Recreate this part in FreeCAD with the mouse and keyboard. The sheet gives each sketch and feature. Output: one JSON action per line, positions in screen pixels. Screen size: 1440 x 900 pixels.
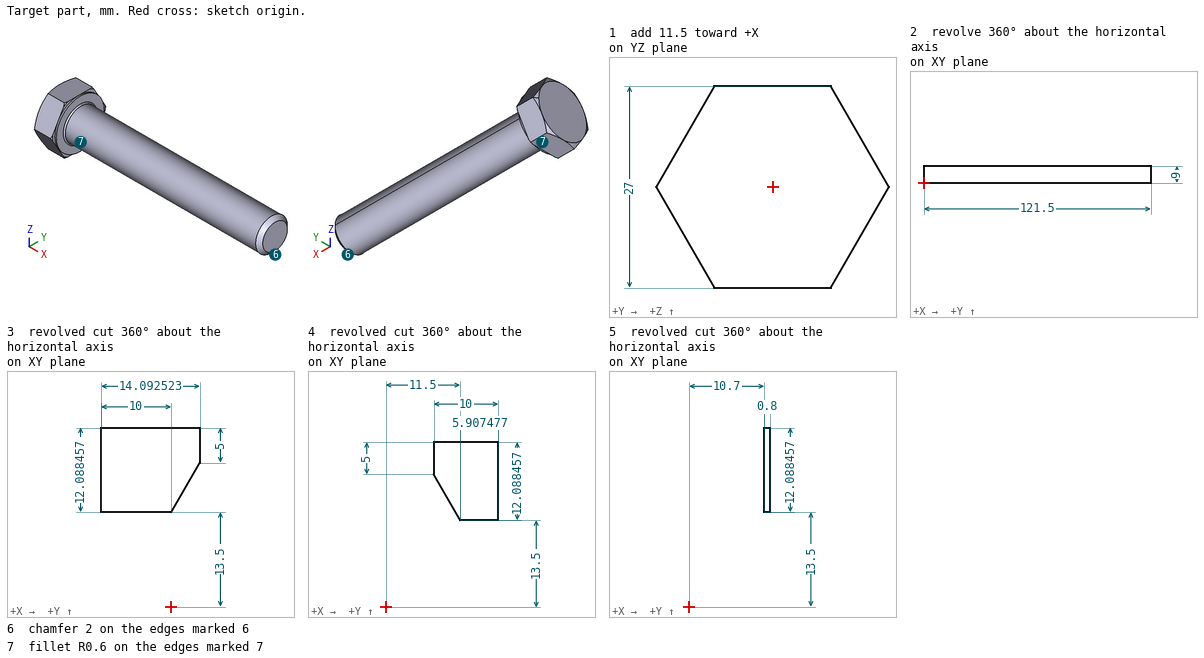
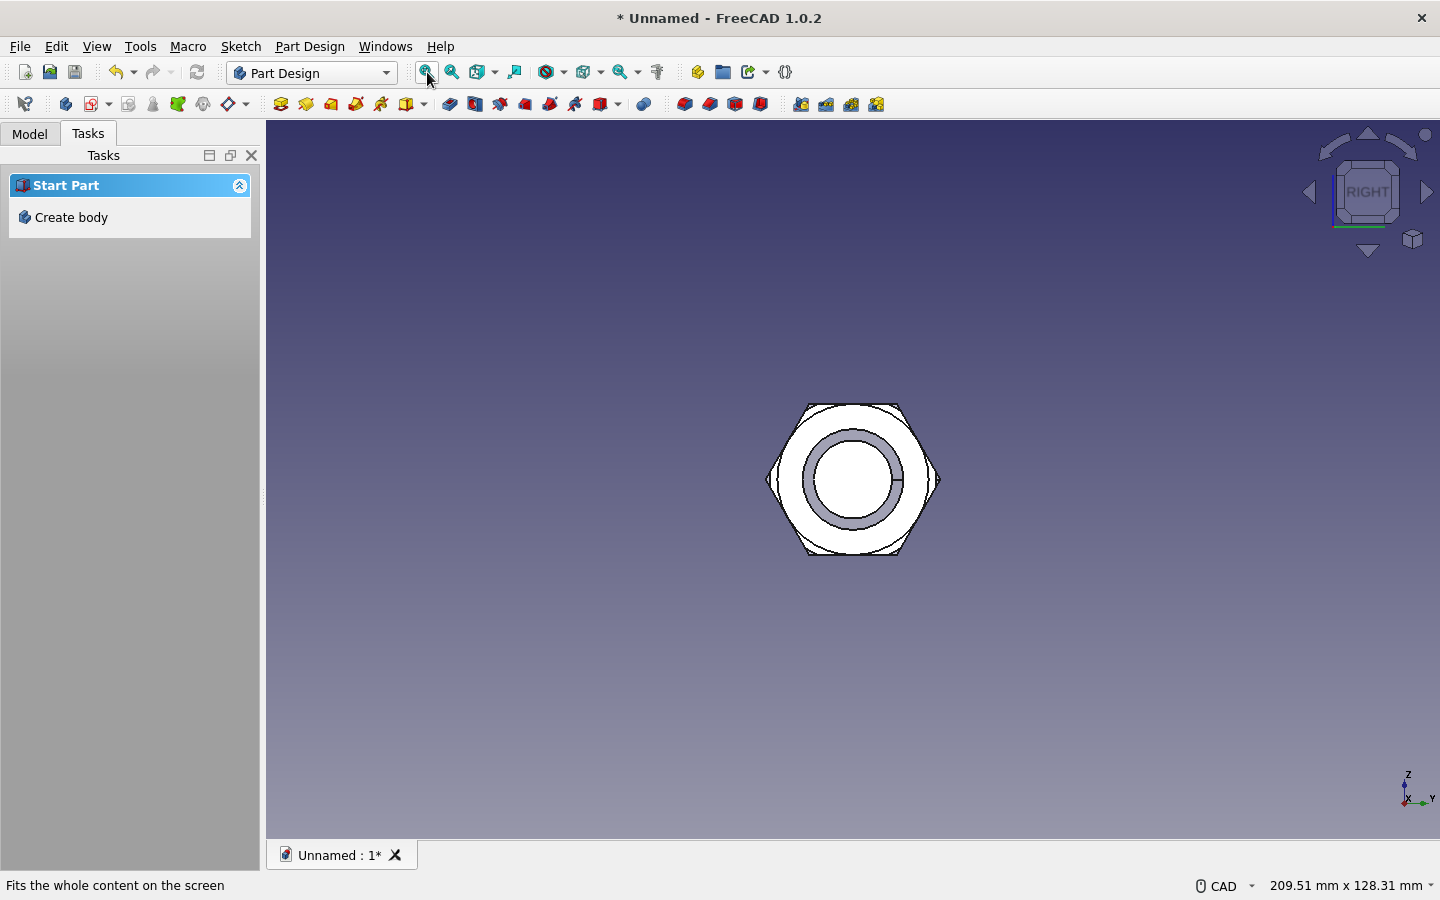
{"action": "key", "text": "5"}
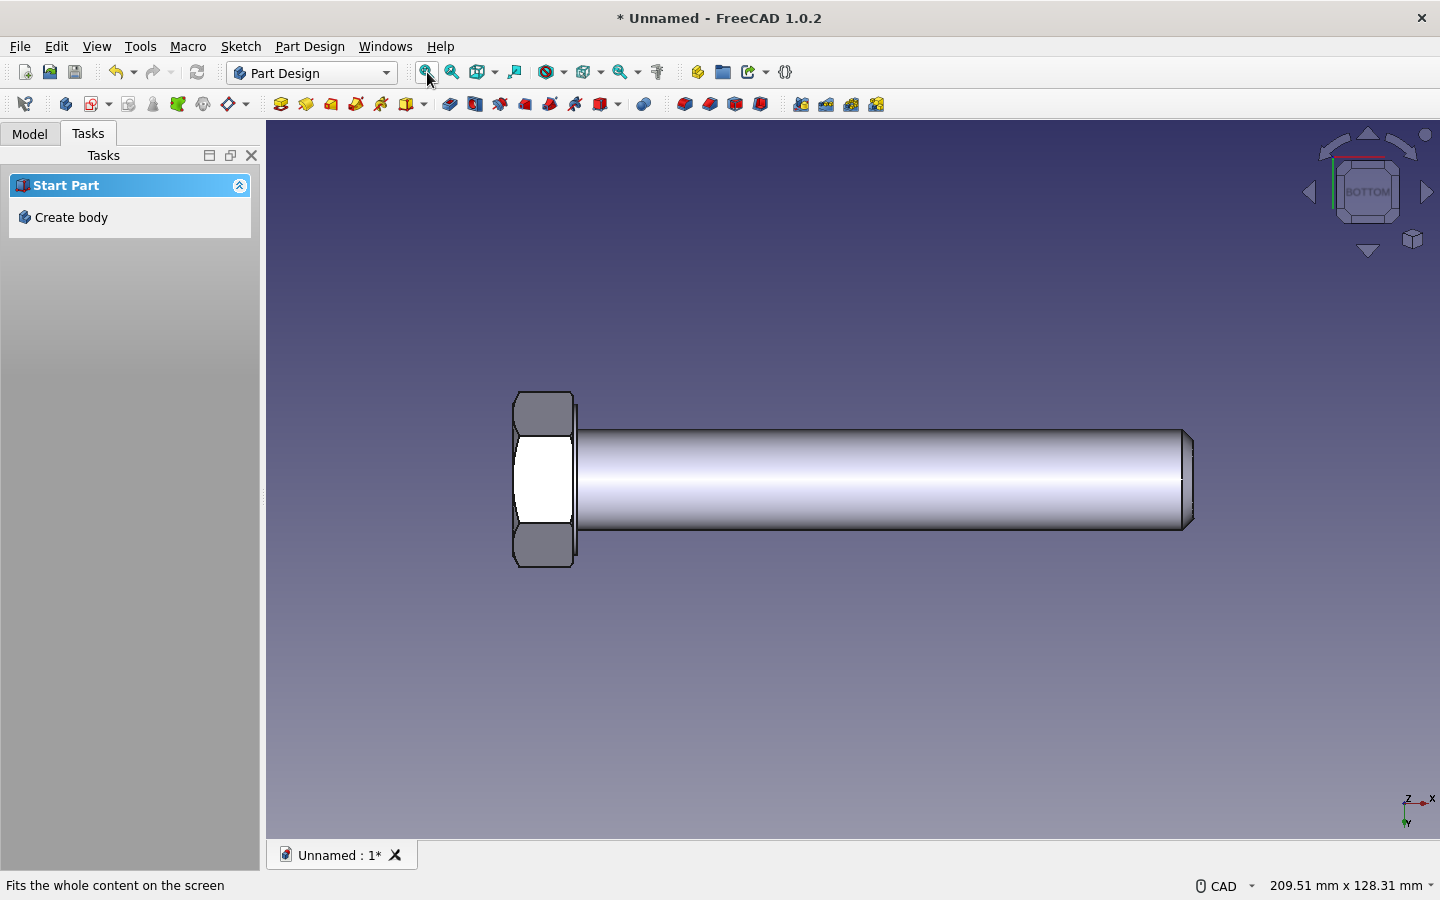
{"action": "key", "text": "4"}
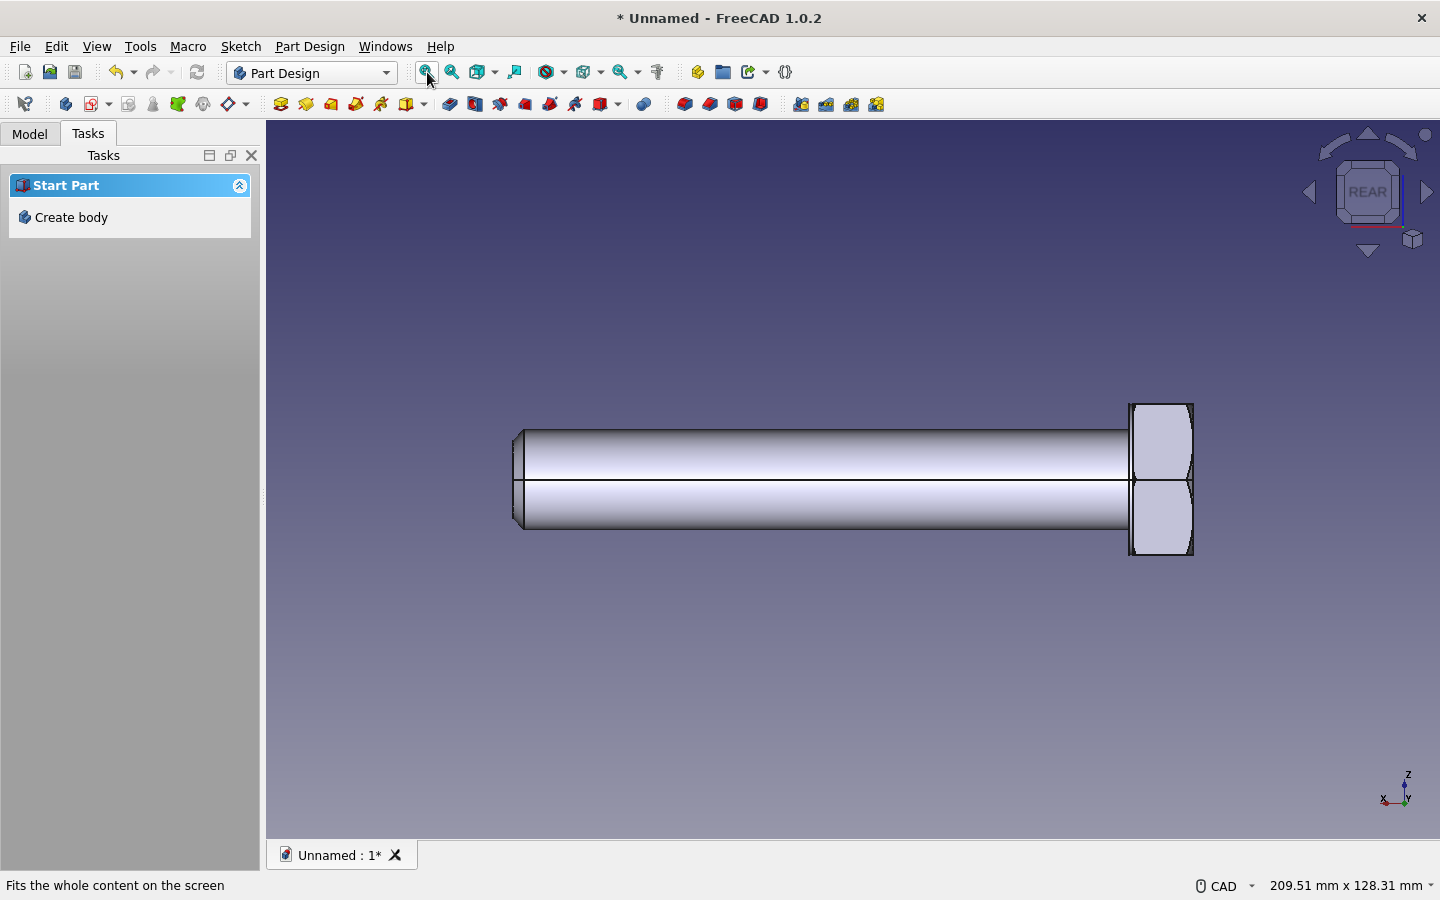
{"action": "key", "text": "6"}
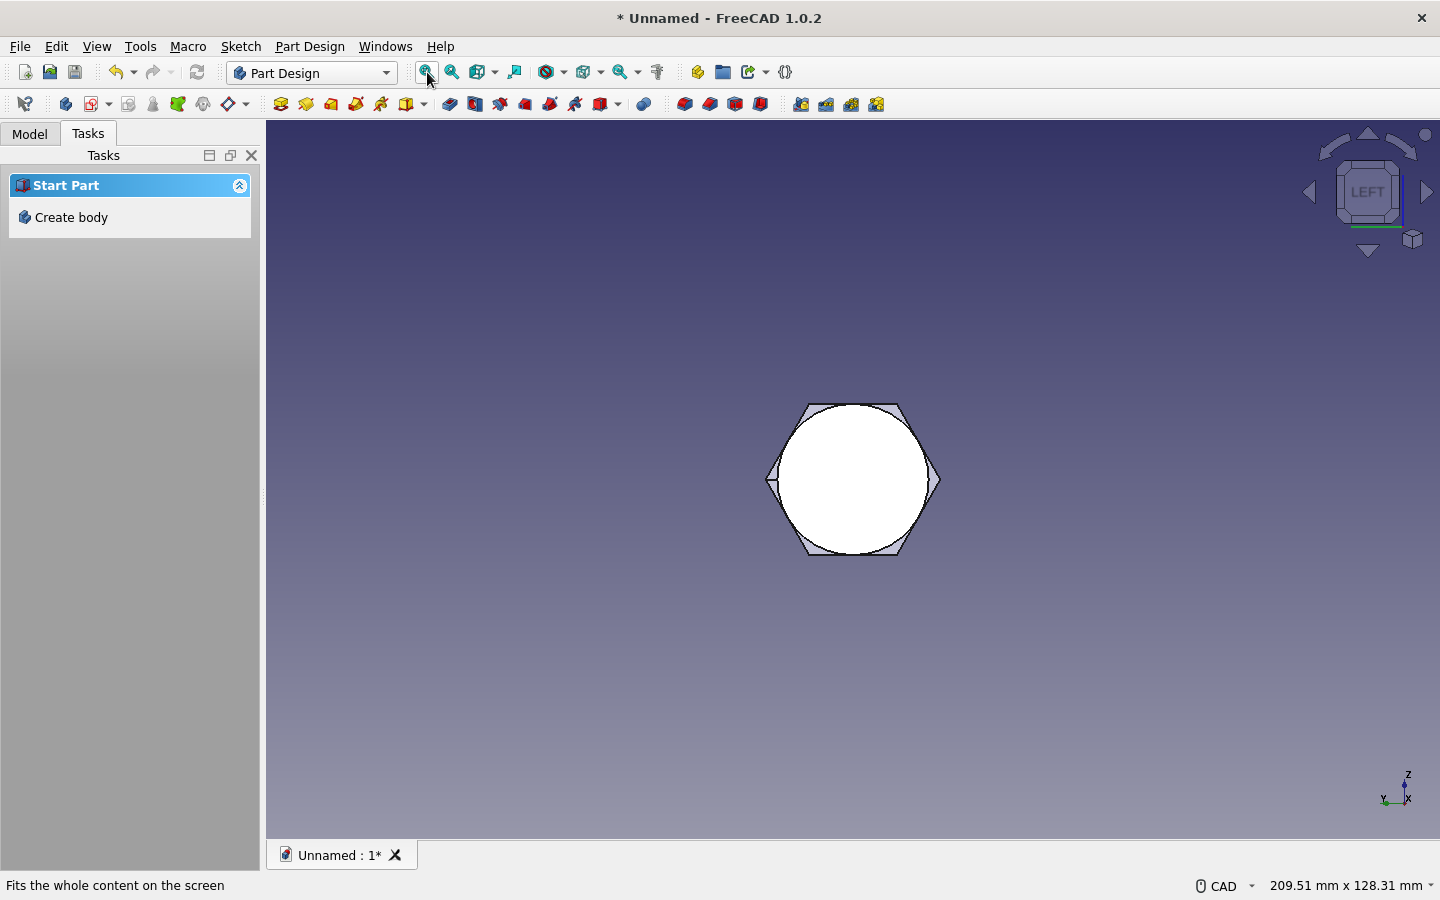
{"action": "left_click", "coordinate": [427, 72]}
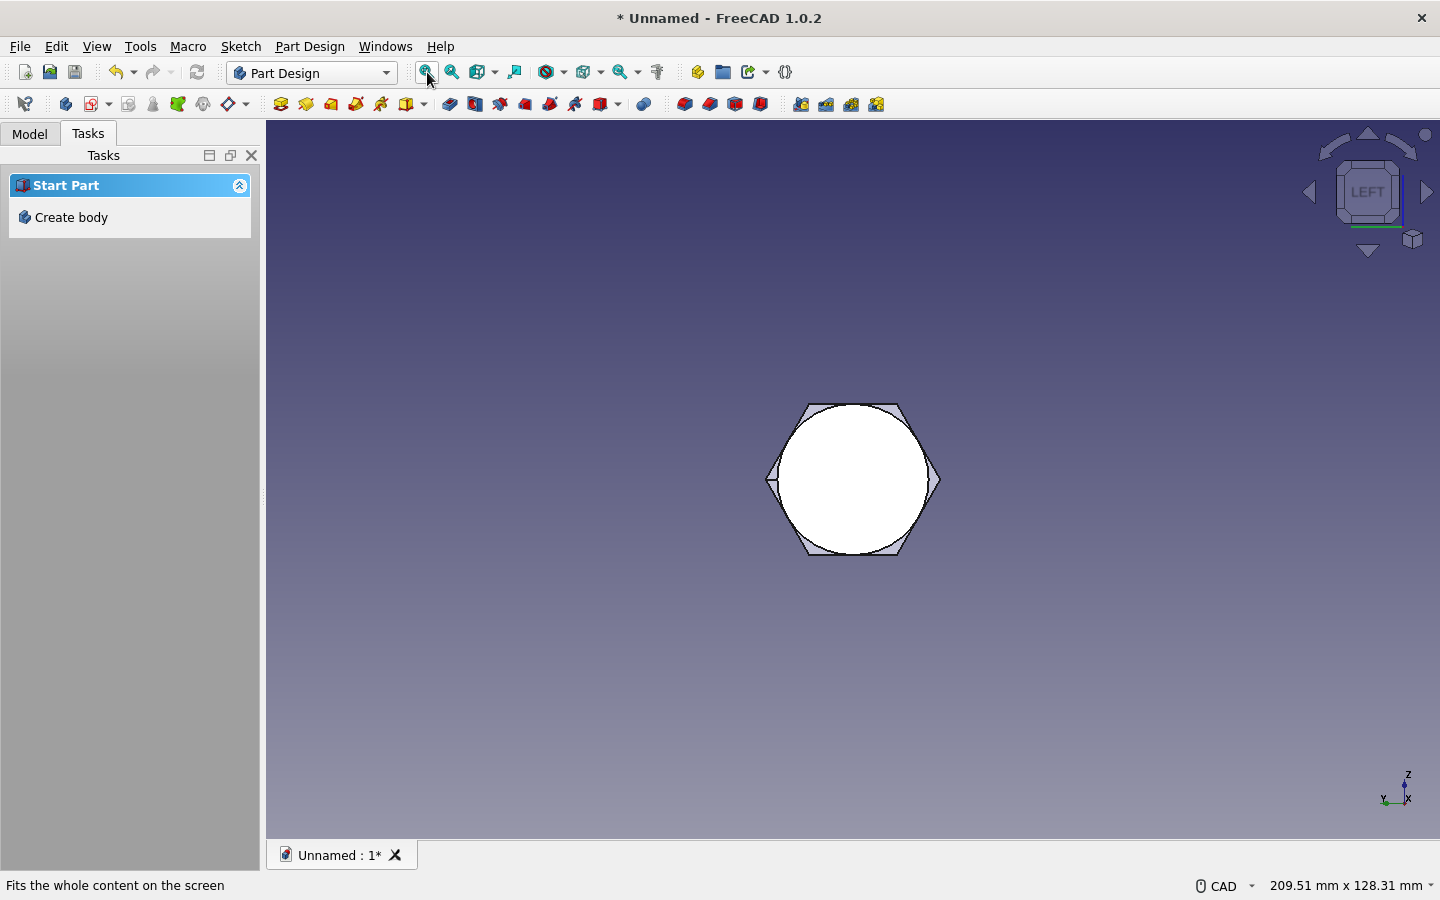
{"action": "key", "text": "v 3"}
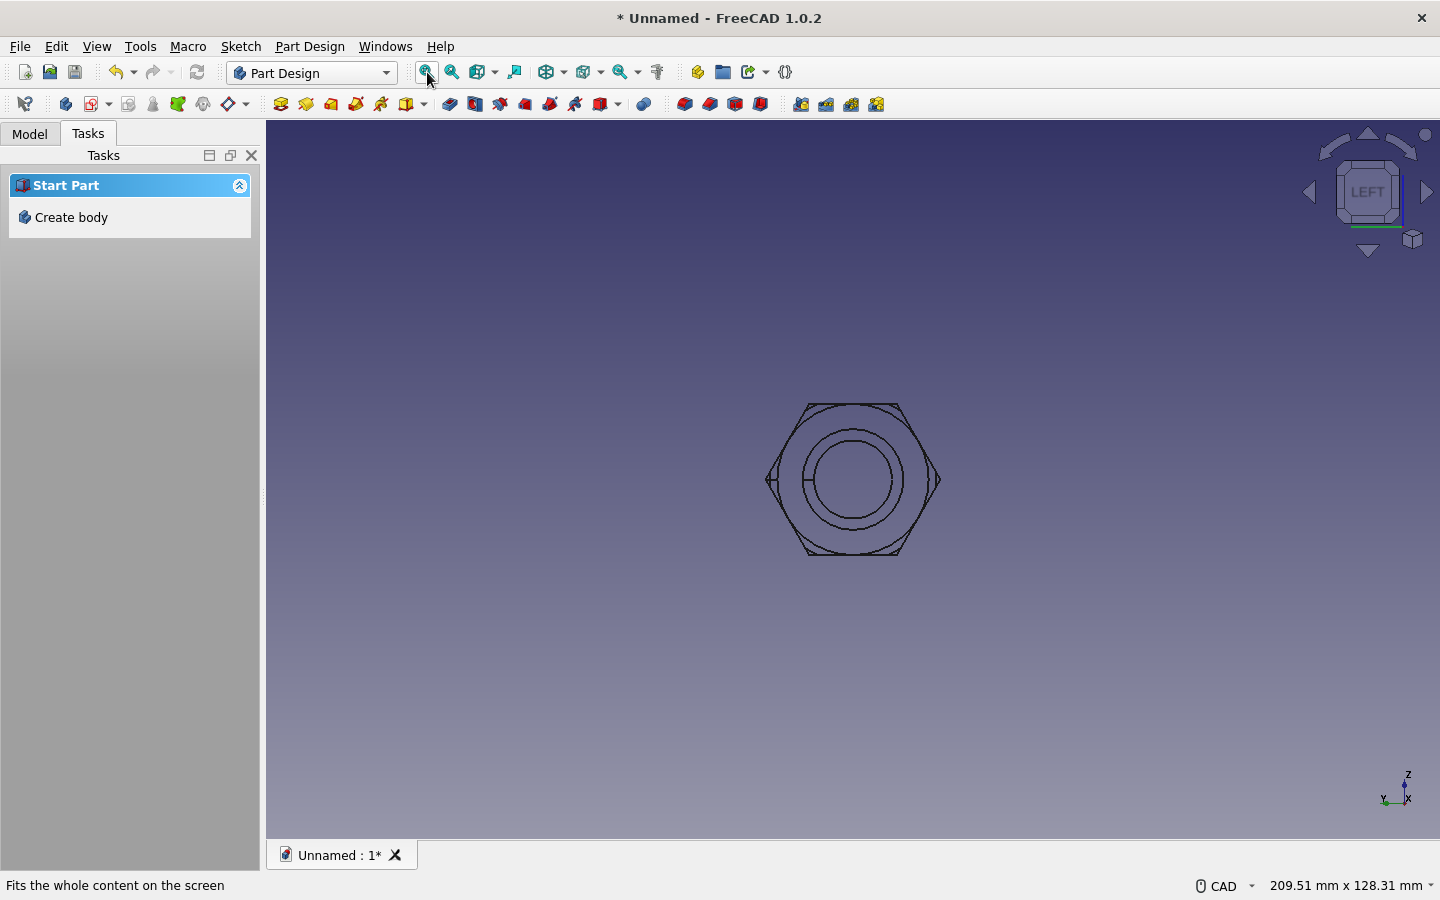
{"action": "key", "text": "0"}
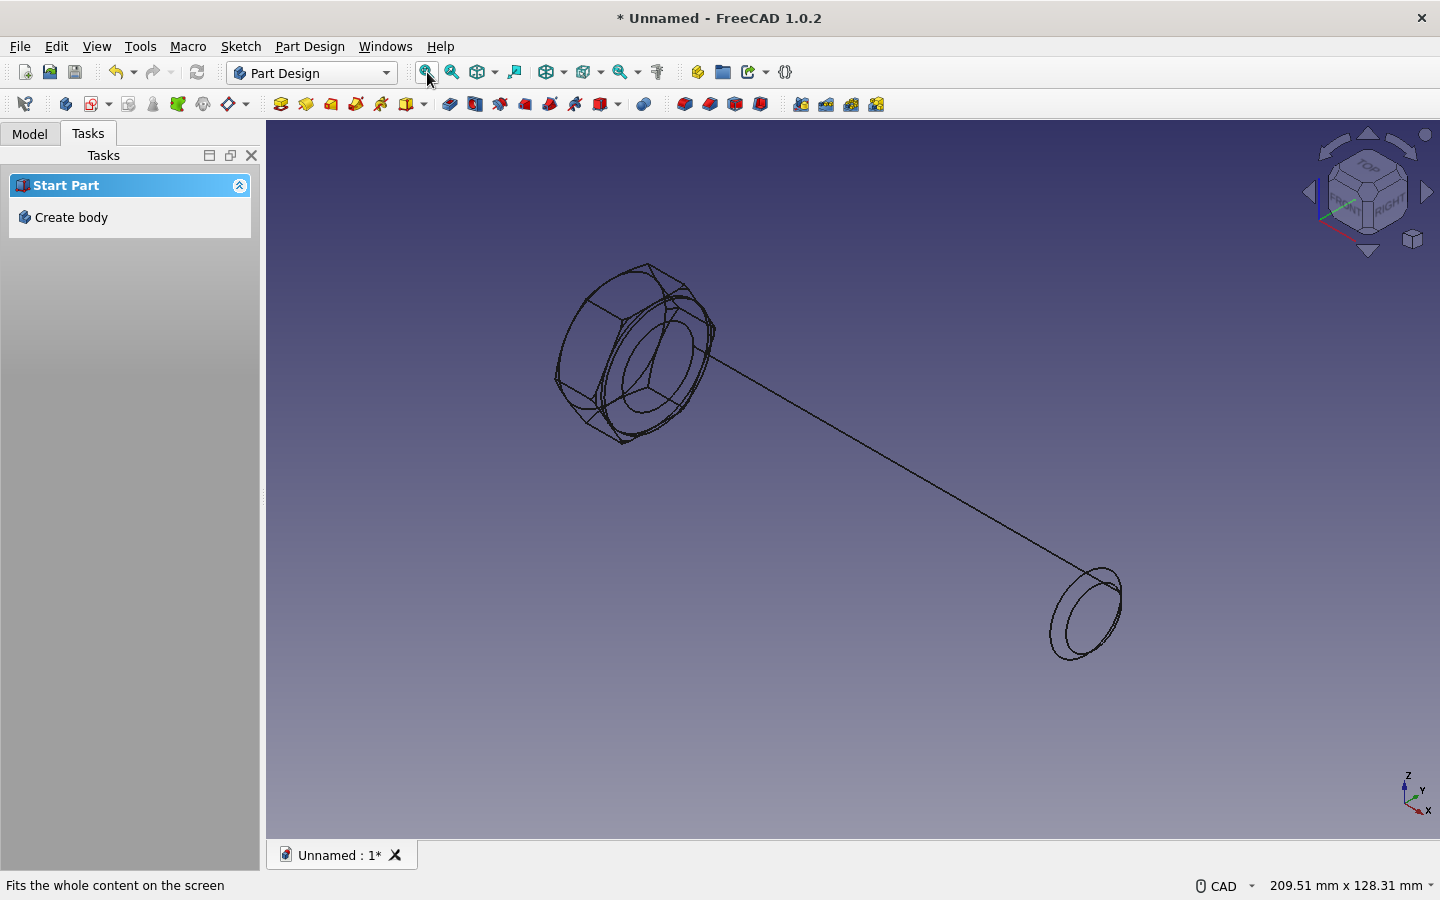
{"action": "left_click", "coordinate": [622, 386]}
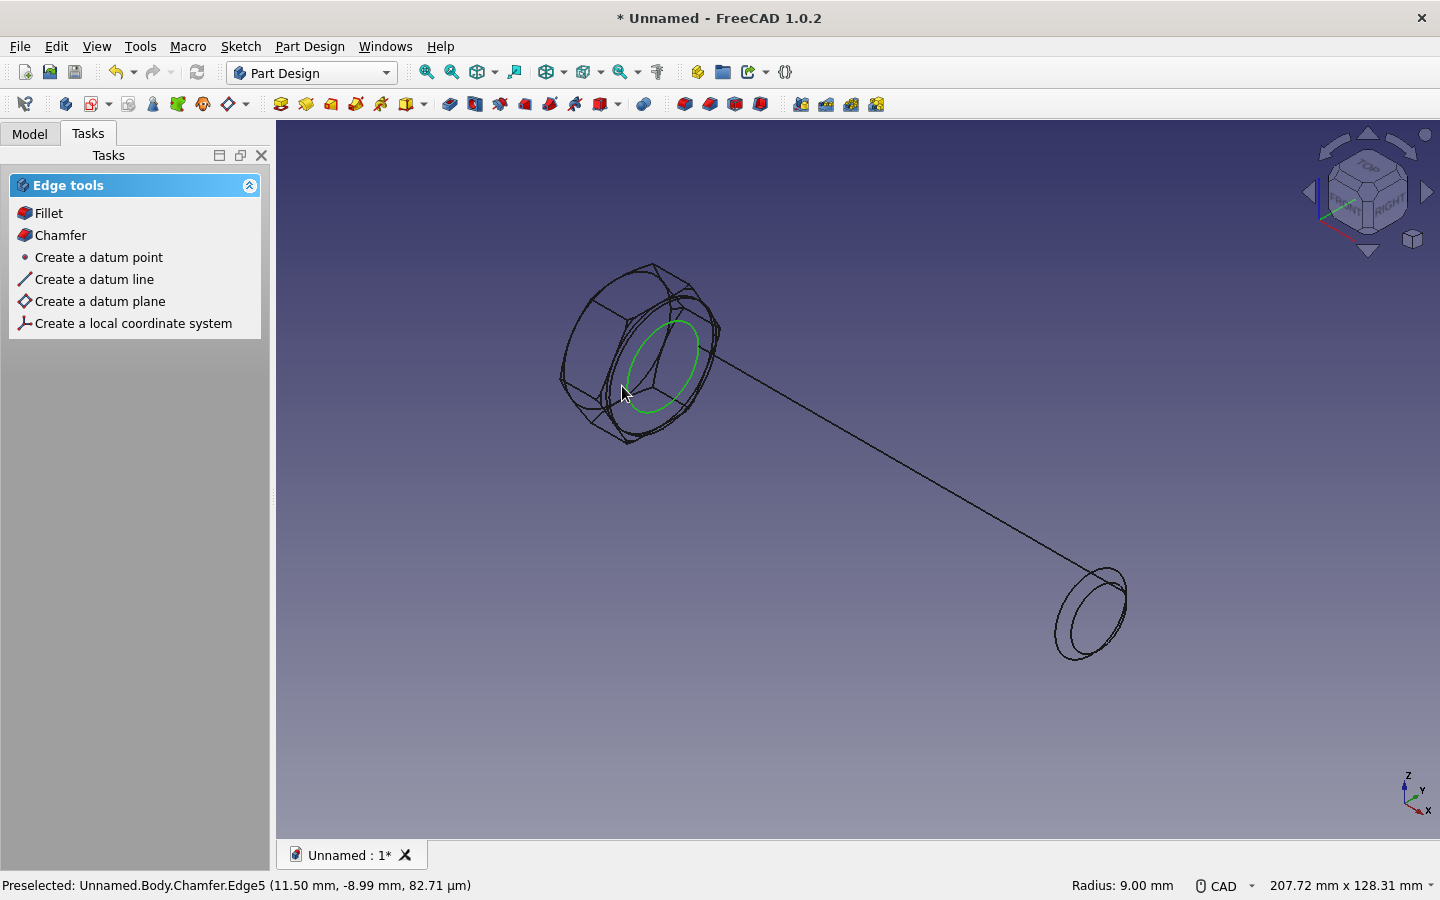
{"action": "key", "text": "v 1"}